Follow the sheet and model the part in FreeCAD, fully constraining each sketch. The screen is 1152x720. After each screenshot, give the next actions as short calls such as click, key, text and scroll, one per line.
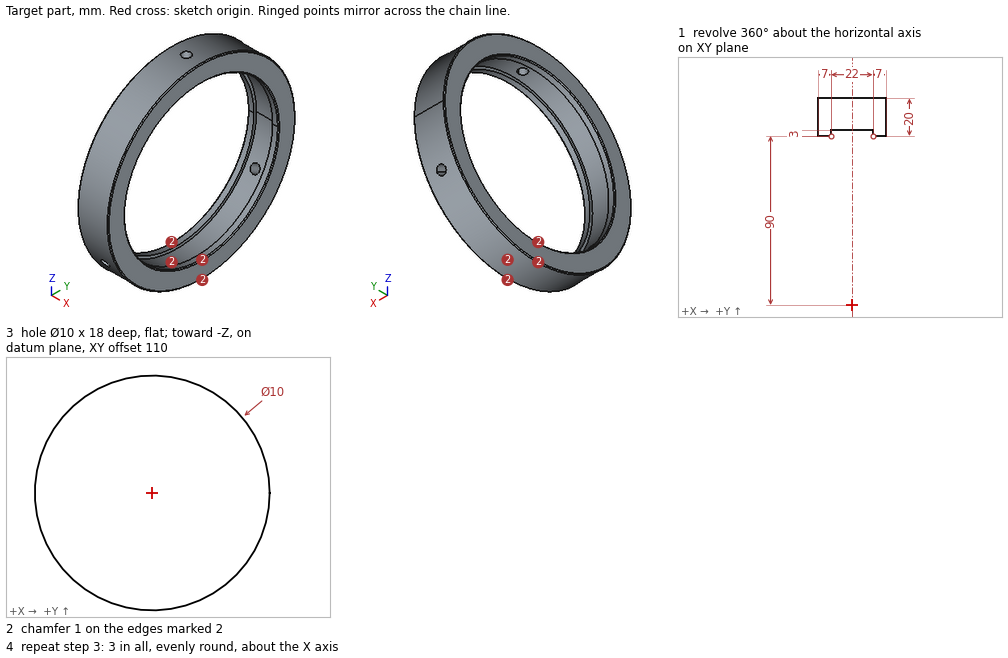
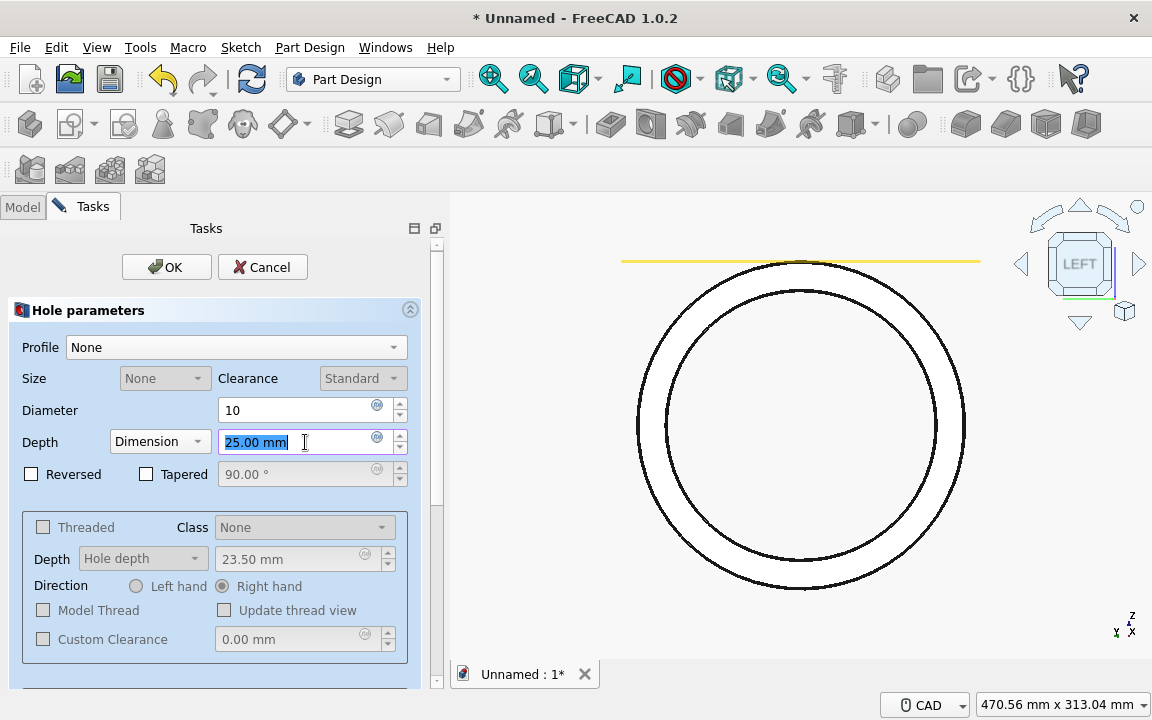
text(18)
key(Tab)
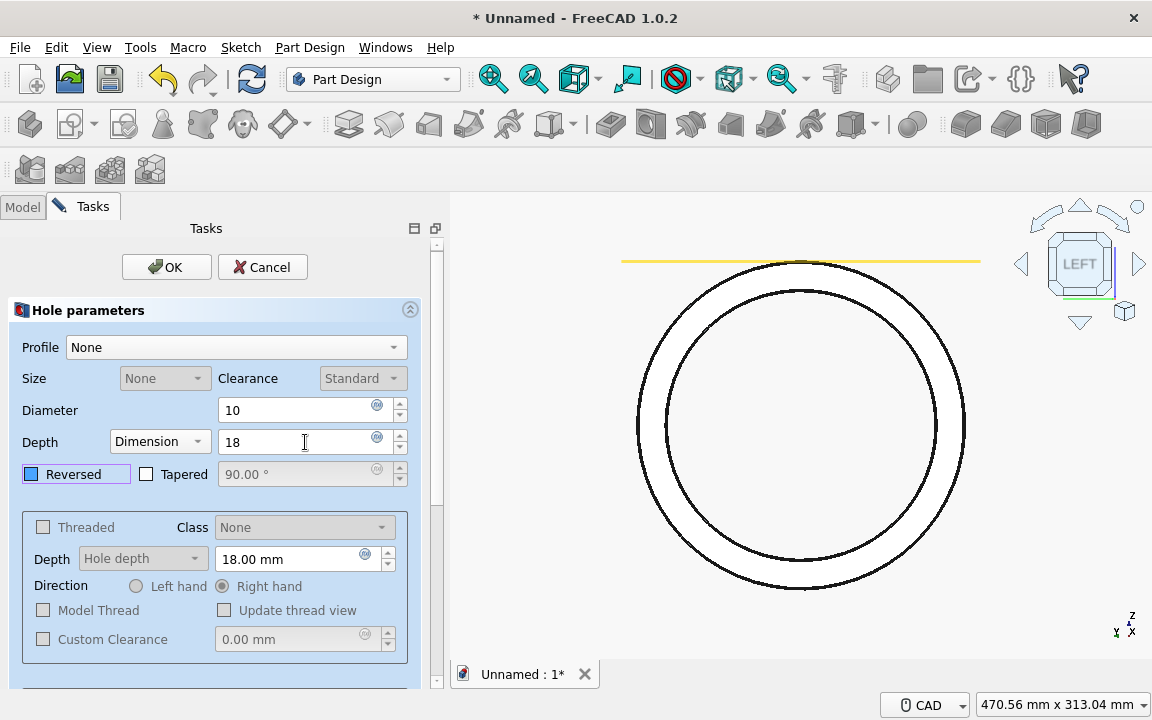
scroll(437, 463, down, 5)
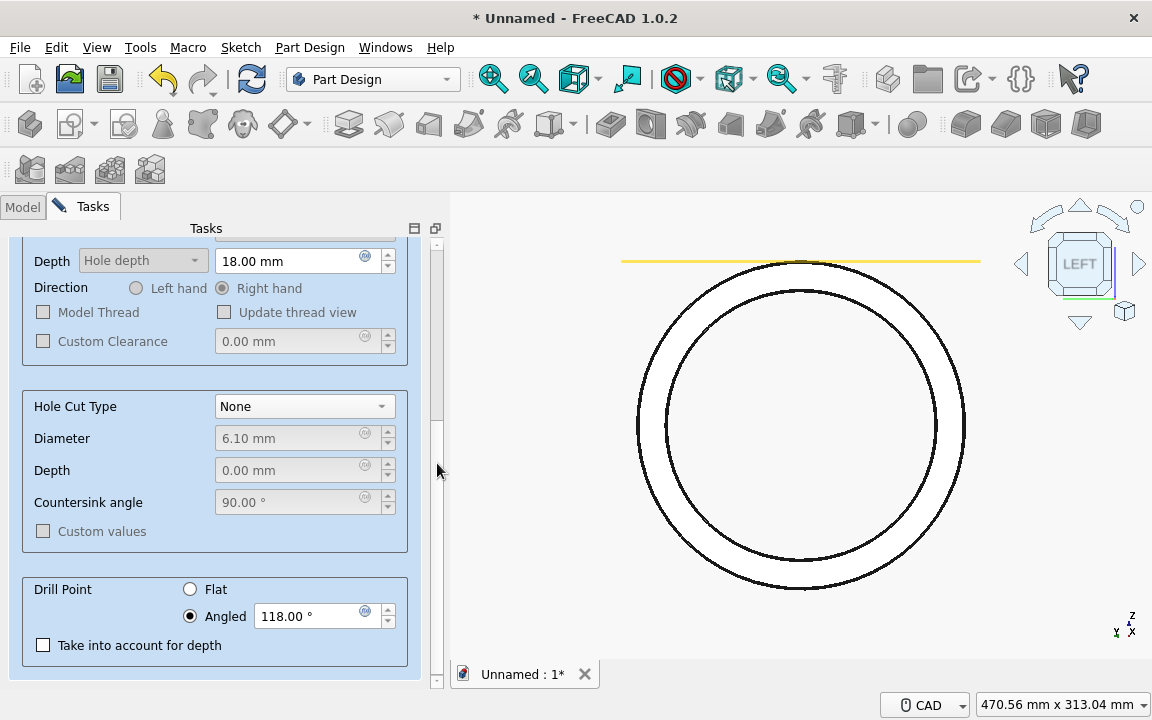
click(191, 589)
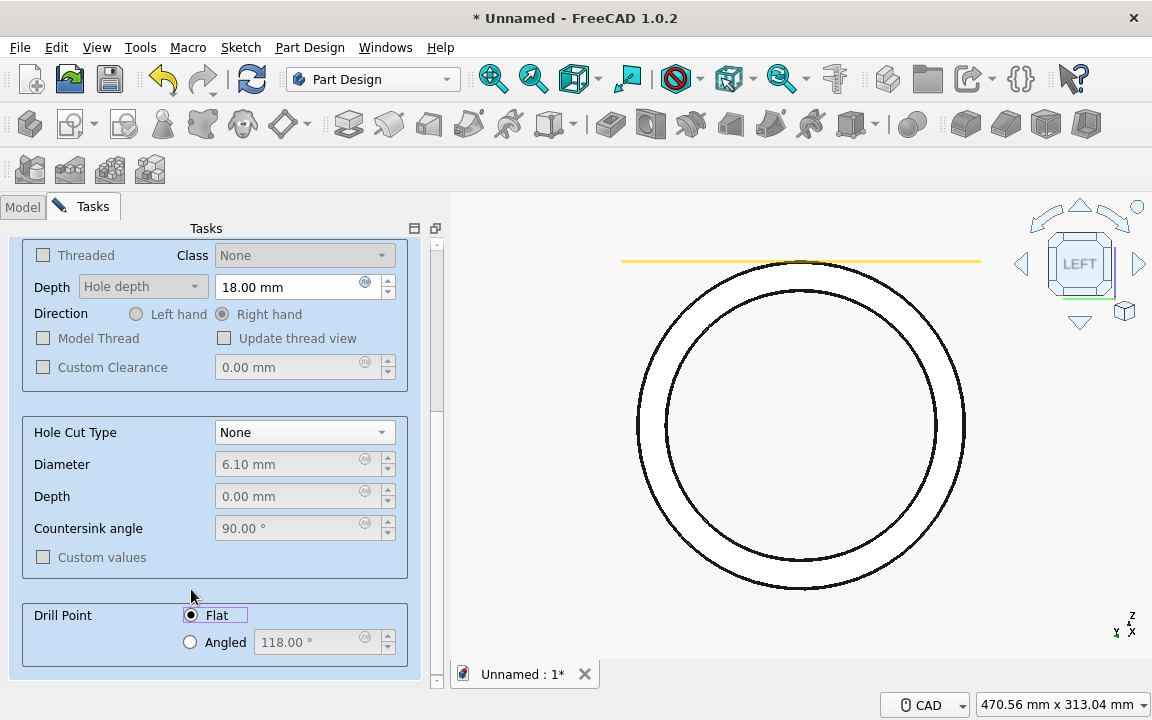
scroll(437, 463, up, 6)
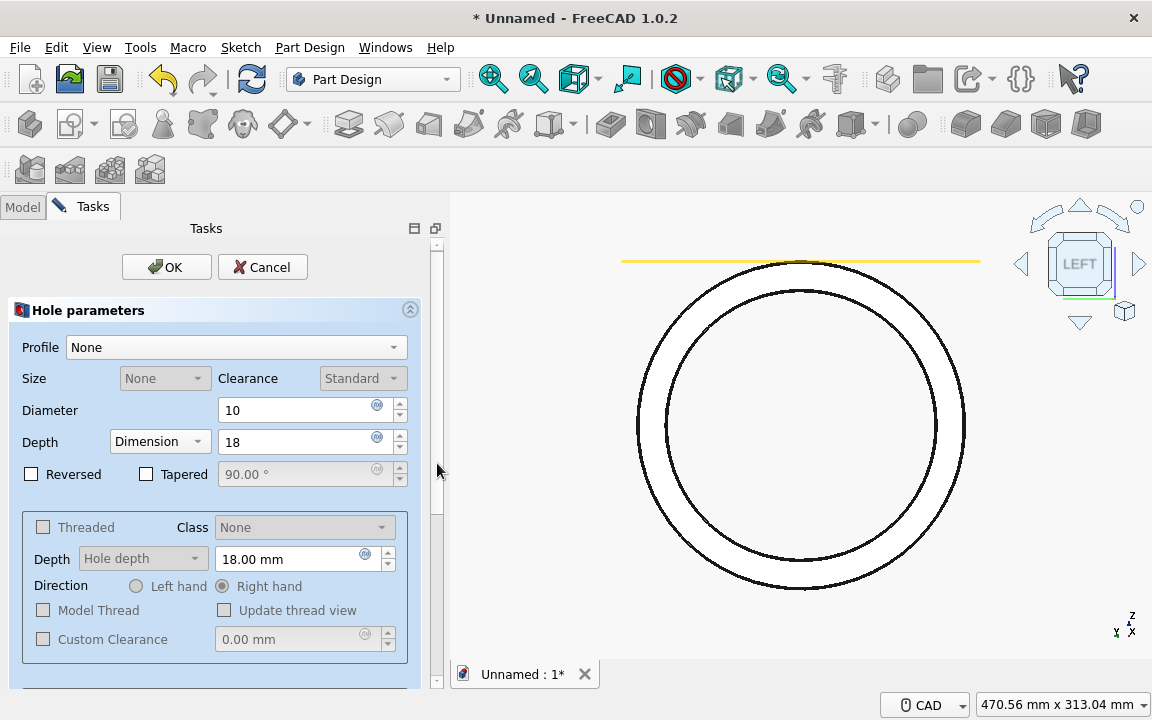
click(167, 267)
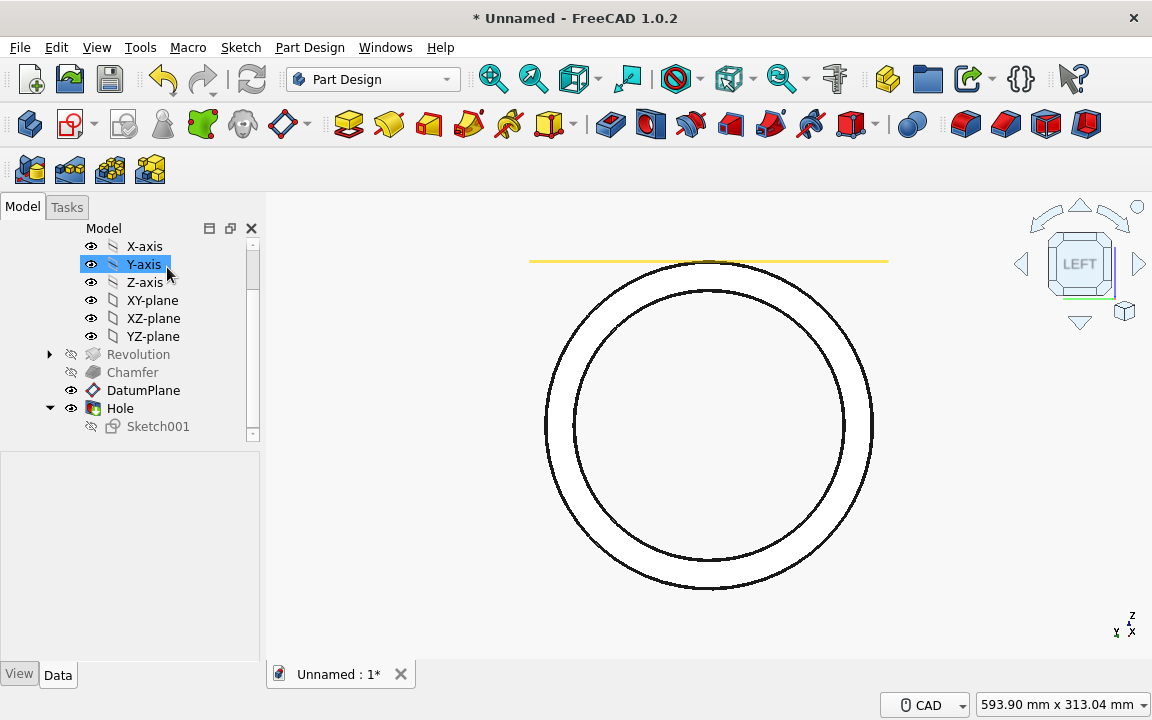
click(116, 390)
key(space)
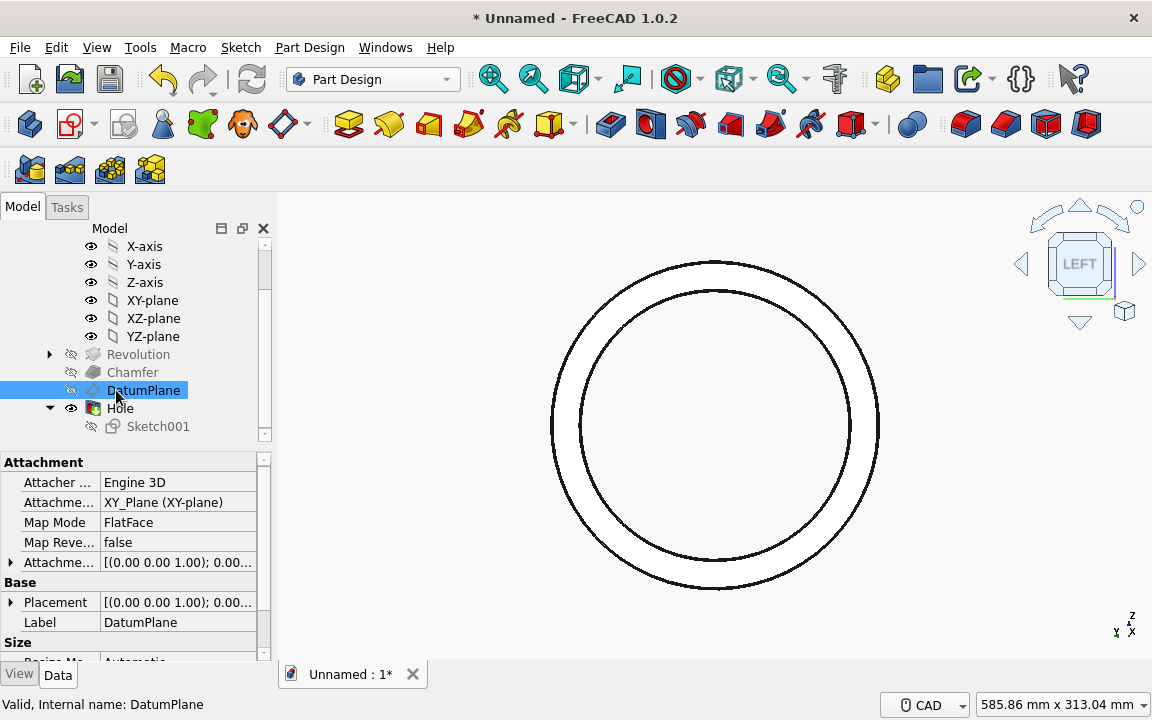
click(116, 408)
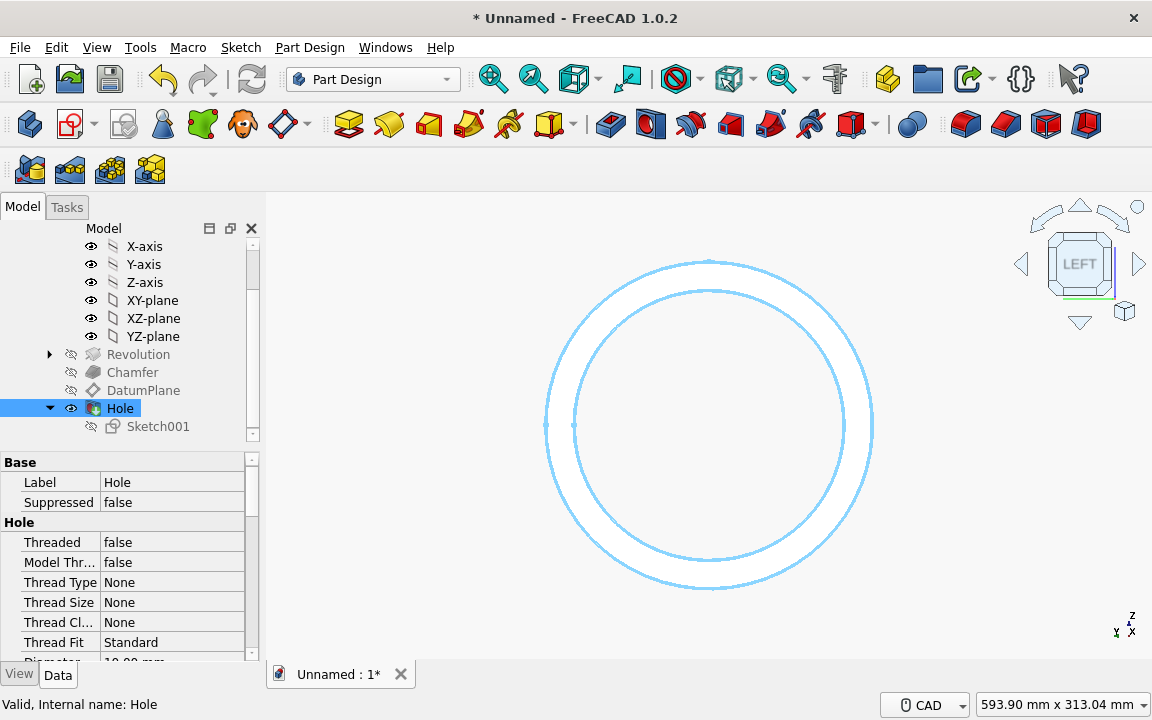
click(110, 170)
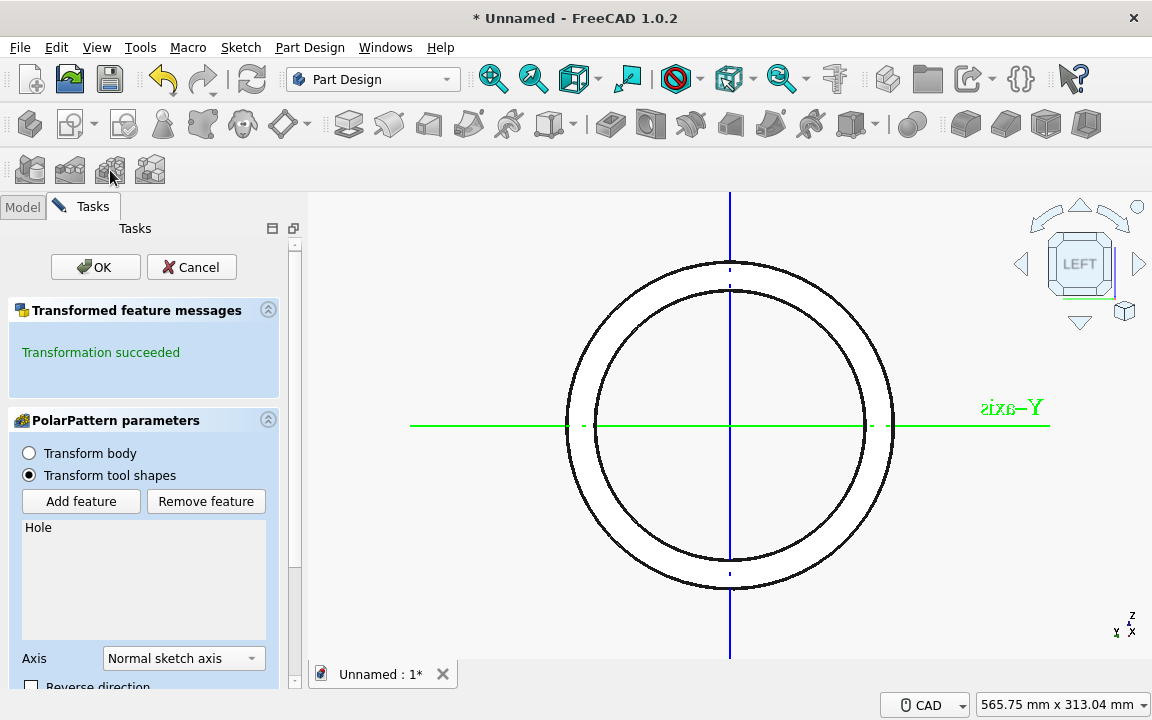
click(184, 658)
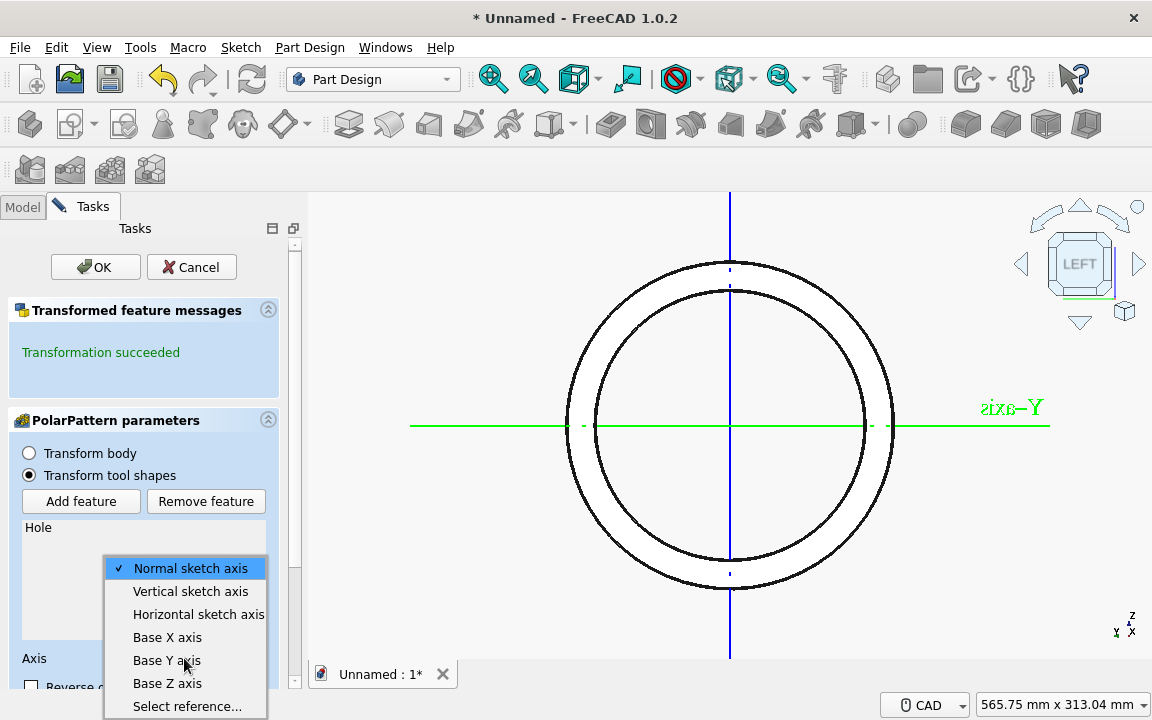
click(184, 638)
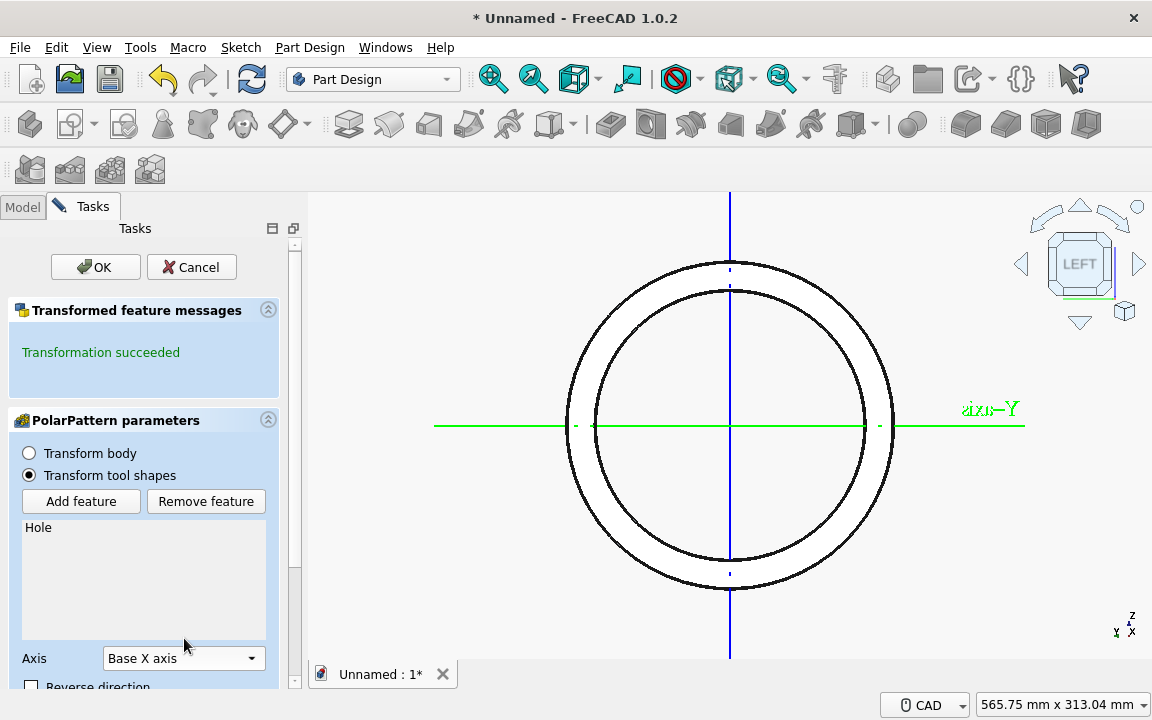
scroll(295, 463, down, 3)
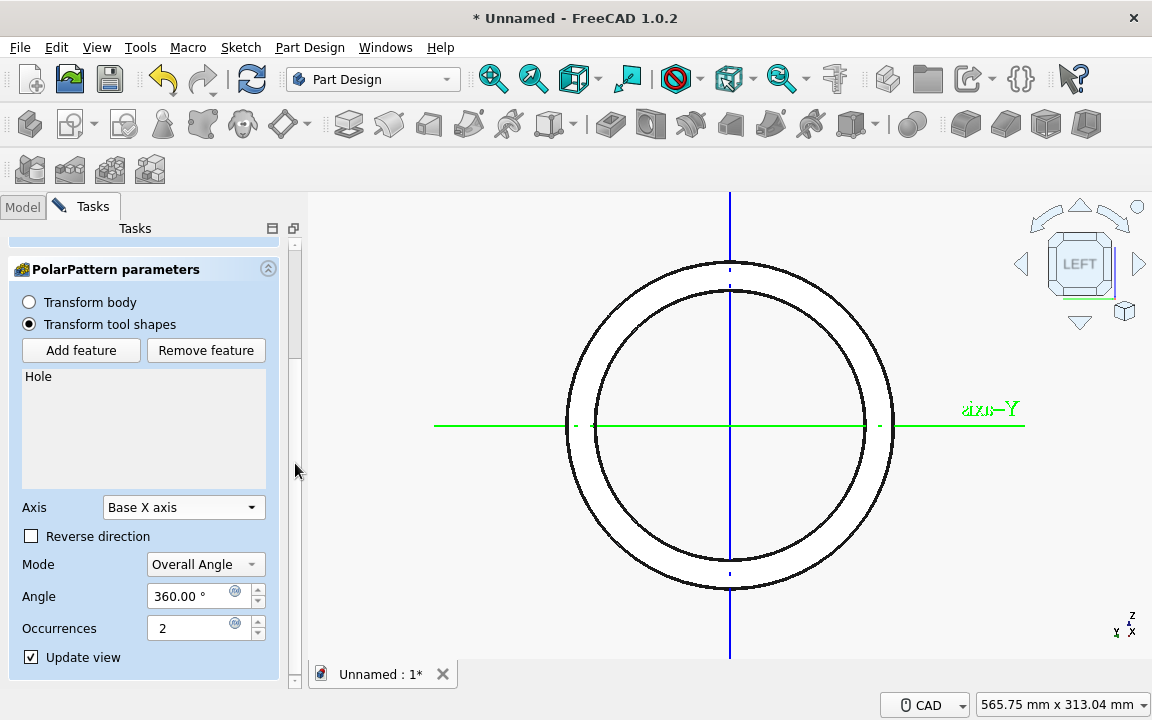
triple_click(198, 628)